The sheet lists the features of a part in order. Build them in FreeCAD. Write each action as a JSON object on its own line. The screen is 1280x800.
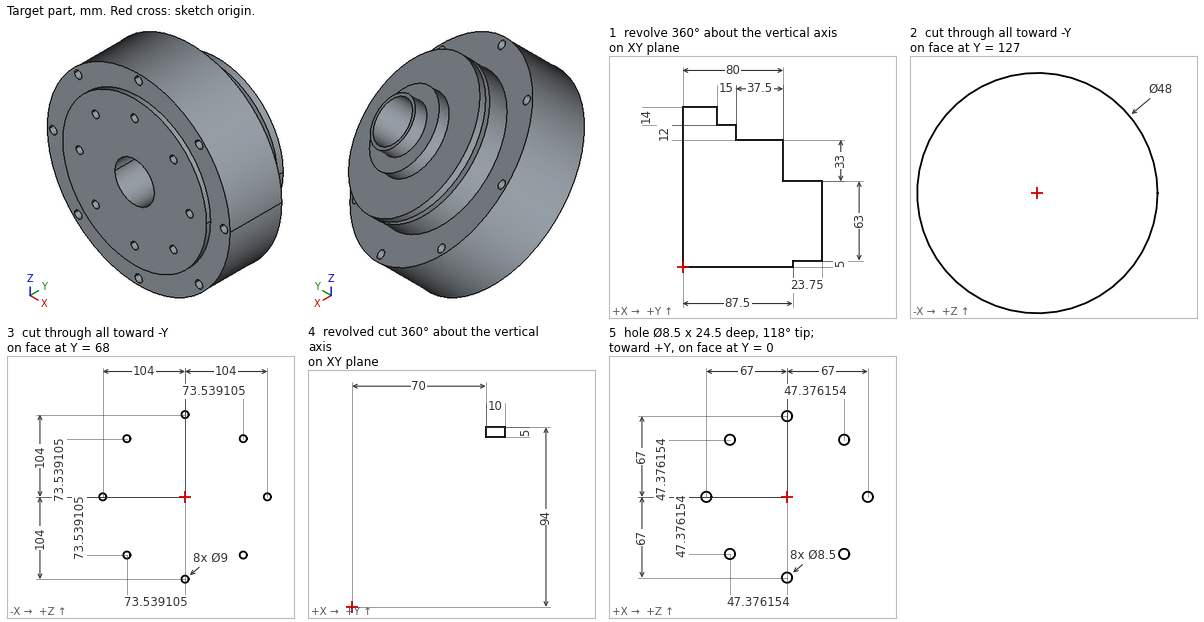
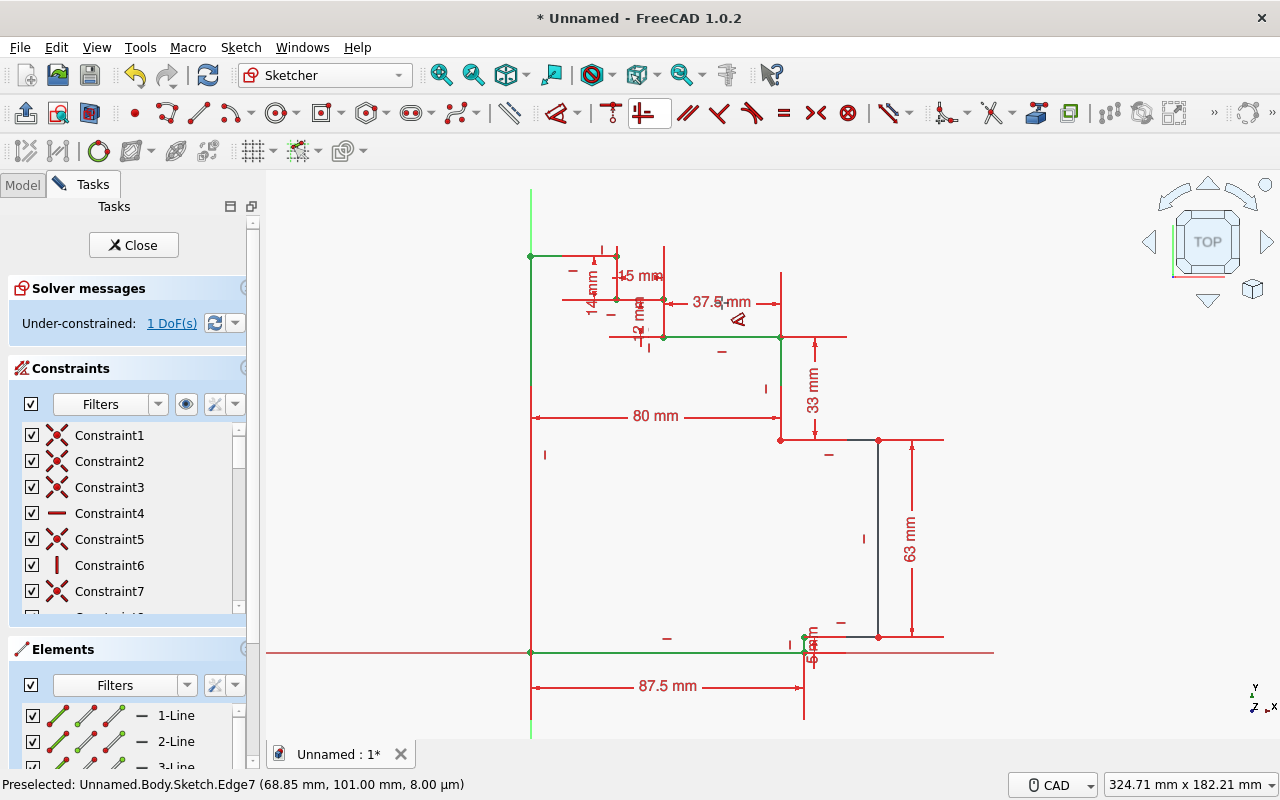
{"action": "left_click", "coordinate": [826, 637]}
{"action": "left_click", "coordinate": [841, 671]}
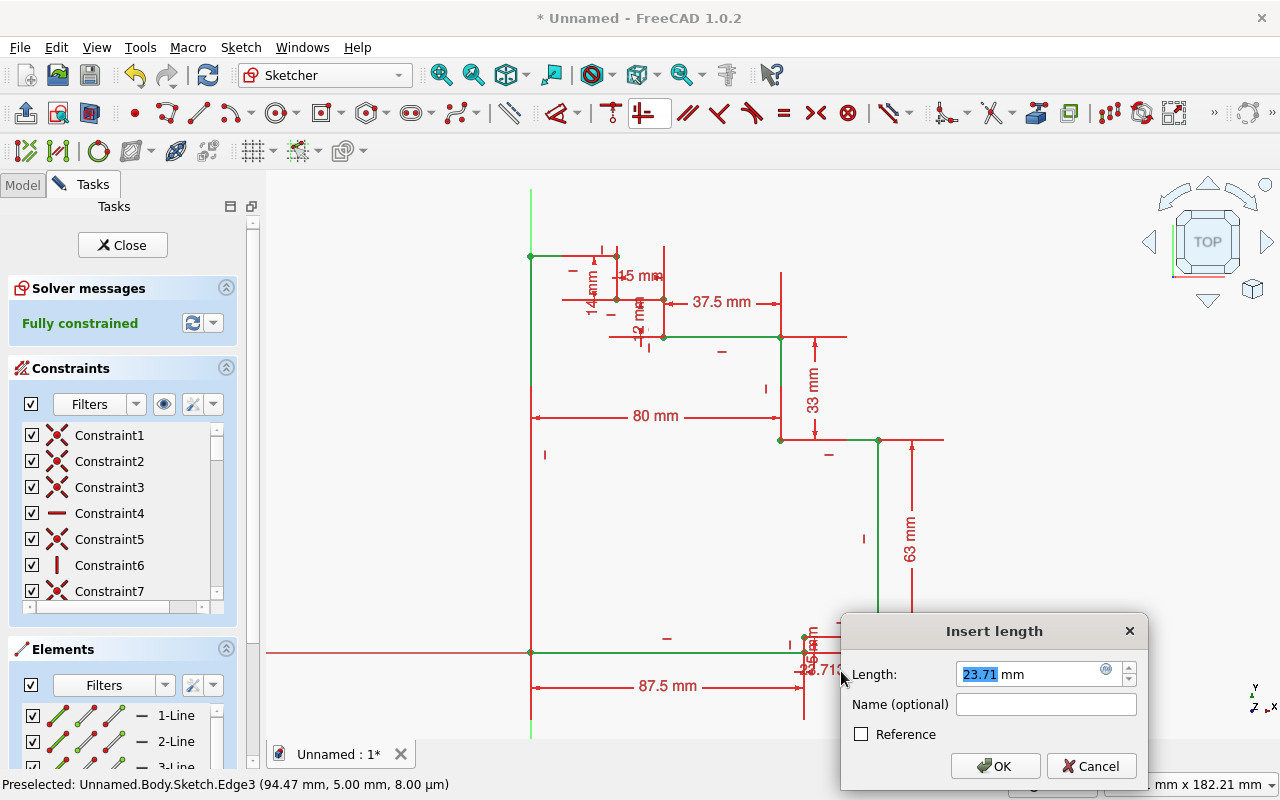
{"action": "type", "text": "23.75"}
{"action": "key", "text": "Return"}
{"action": "key", "text": "Escape"}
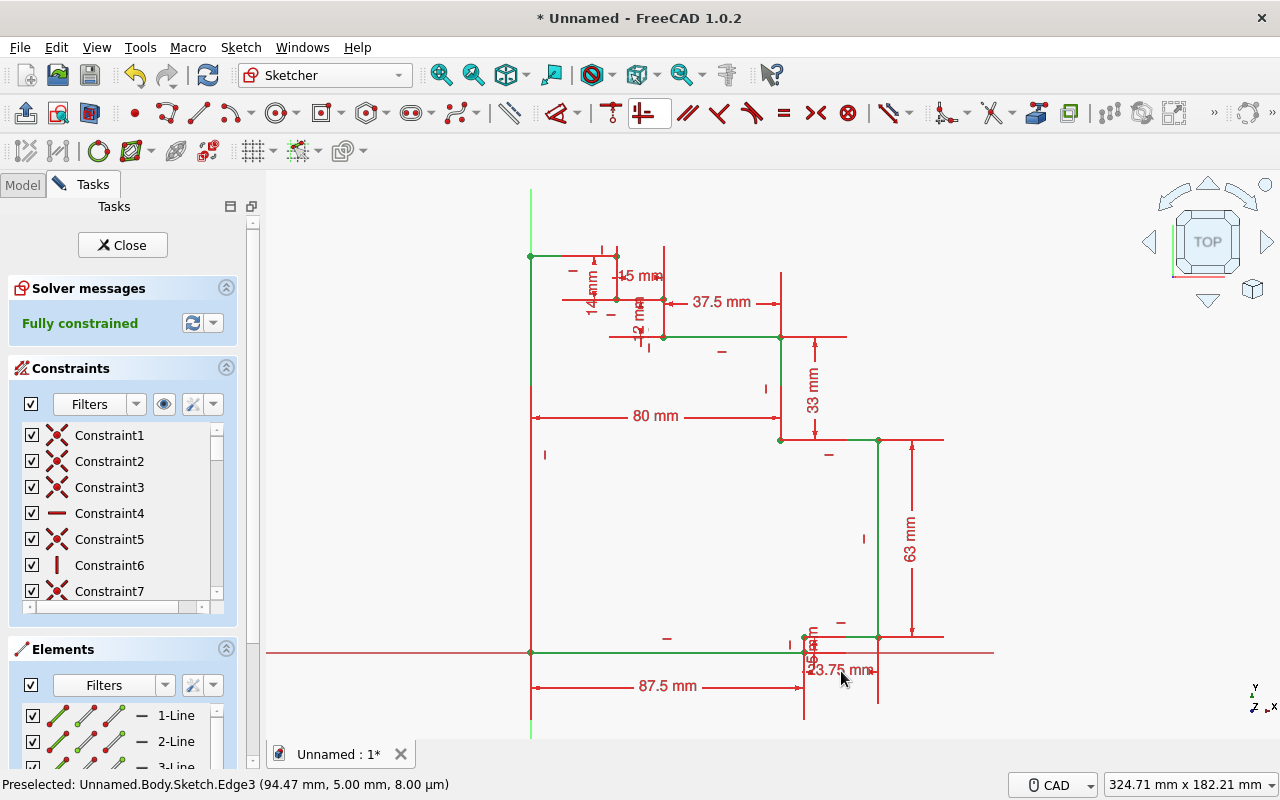
{"action": "left_click", "coordinate": [123, 245]}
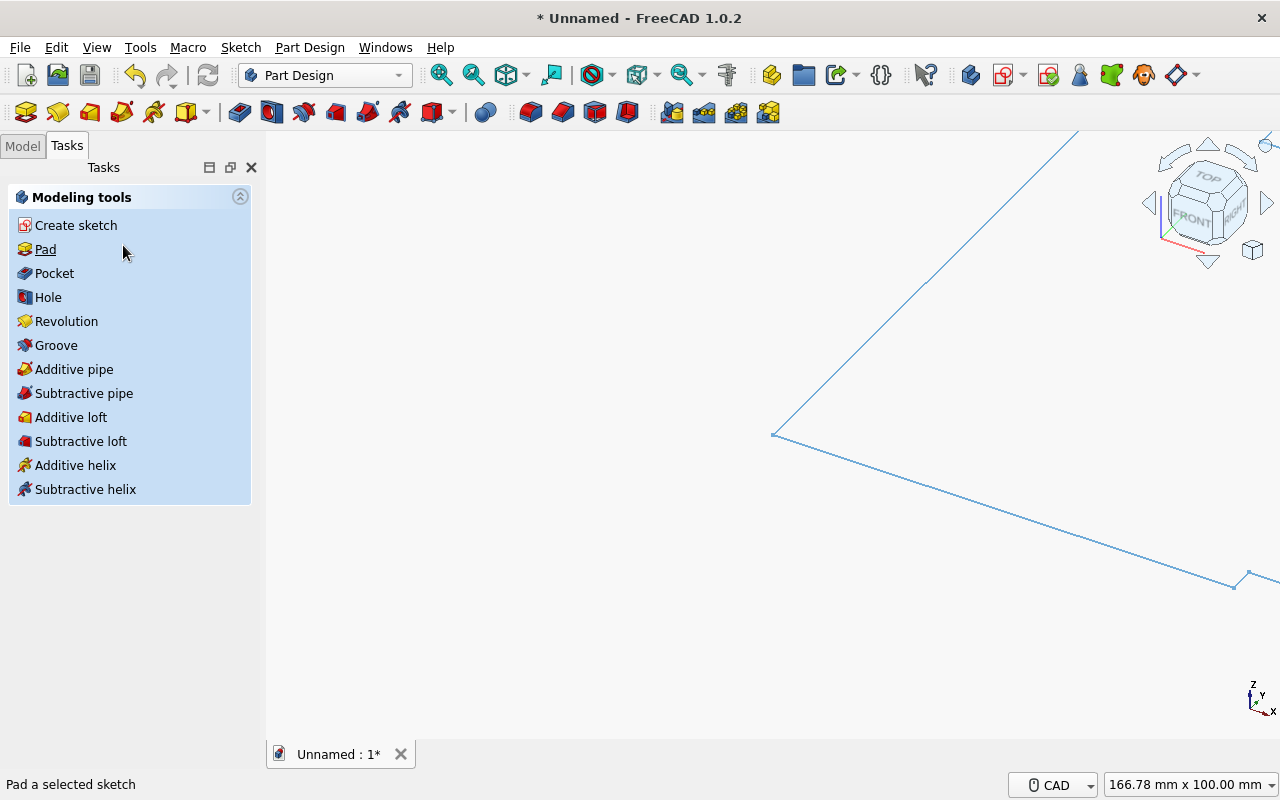
{"action": "left_click", "coordinate": [58, 112]}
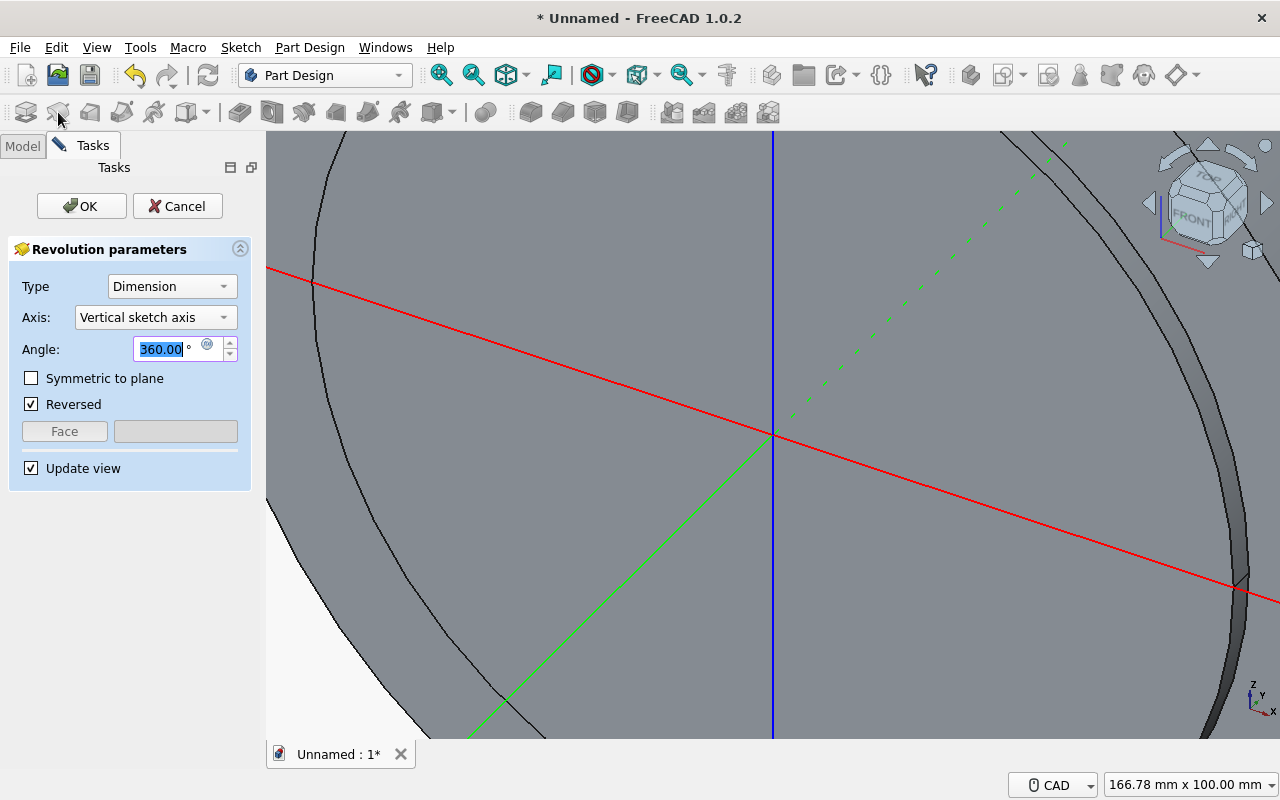
{"action": "left_click", "coordinate": [82, 206]}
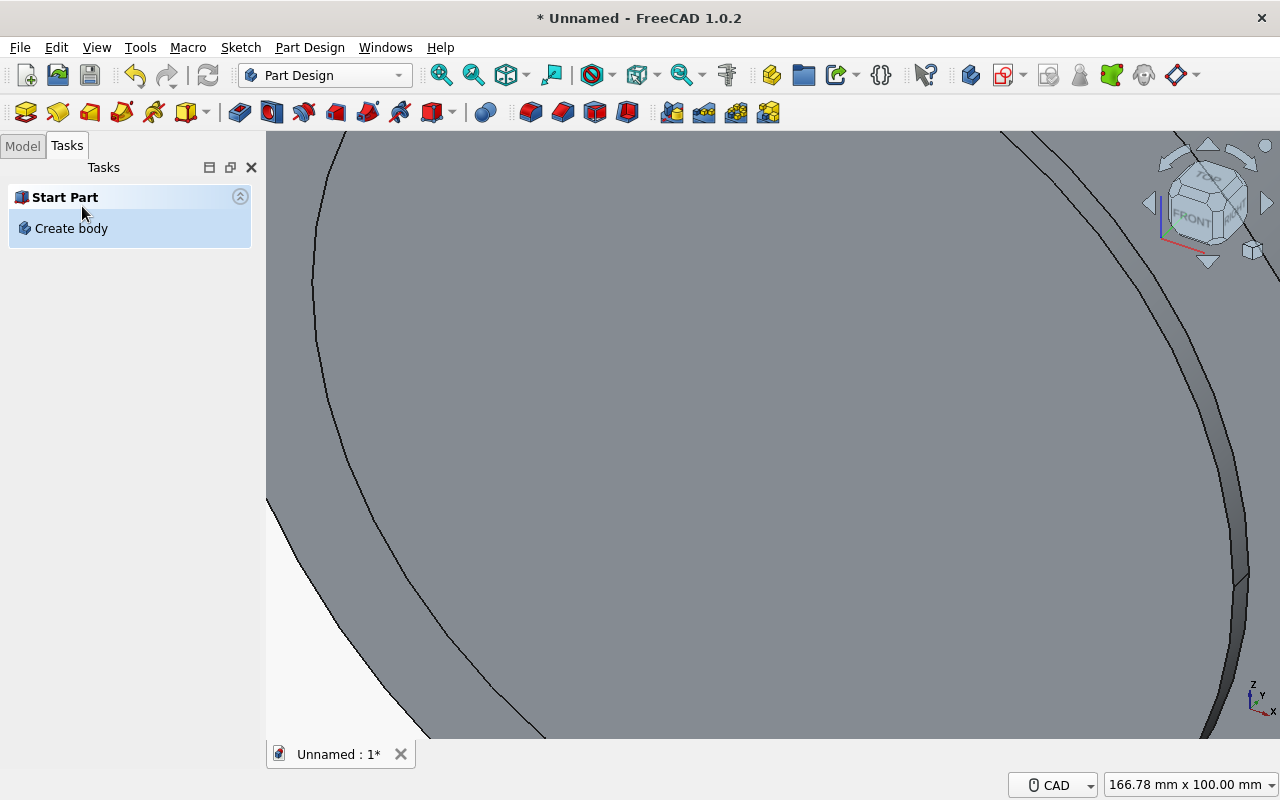
{"action": "left_click", "coordinate": [442, 76]}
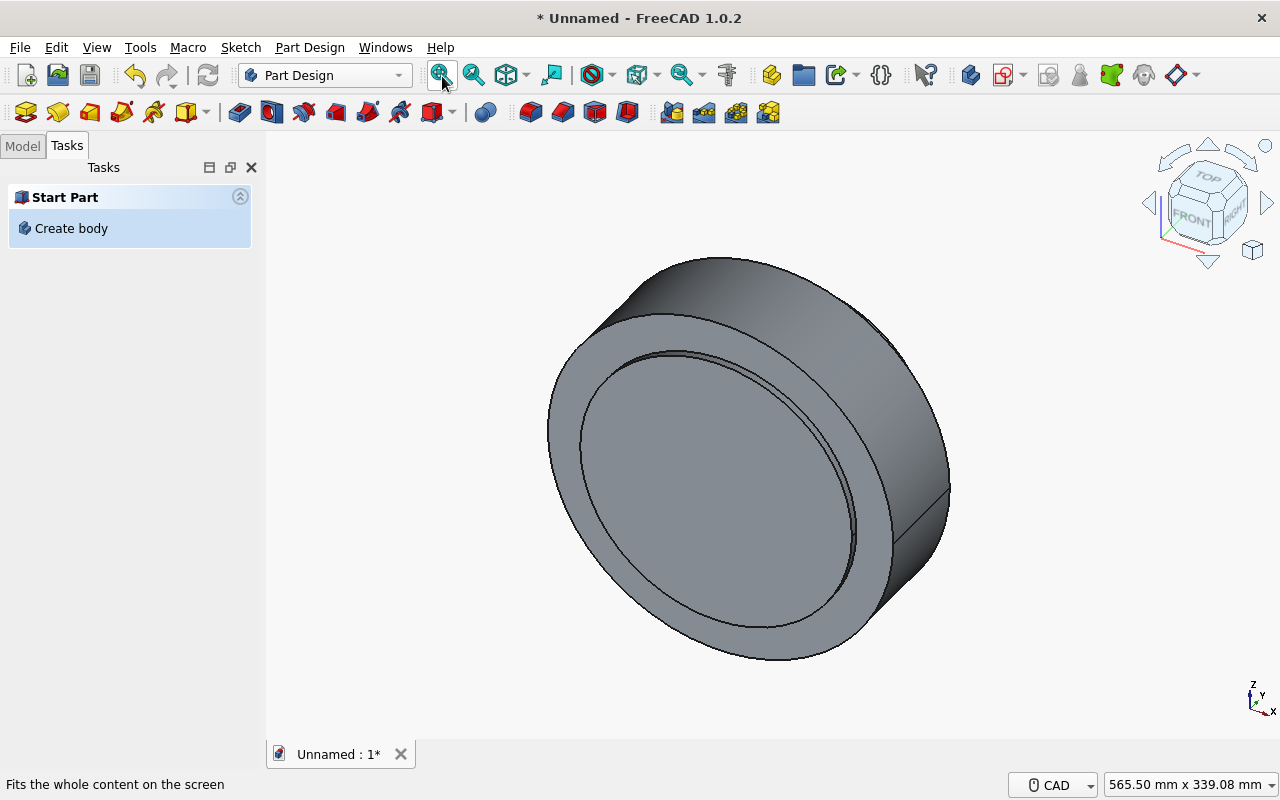
{"action": "key", "text": "4"}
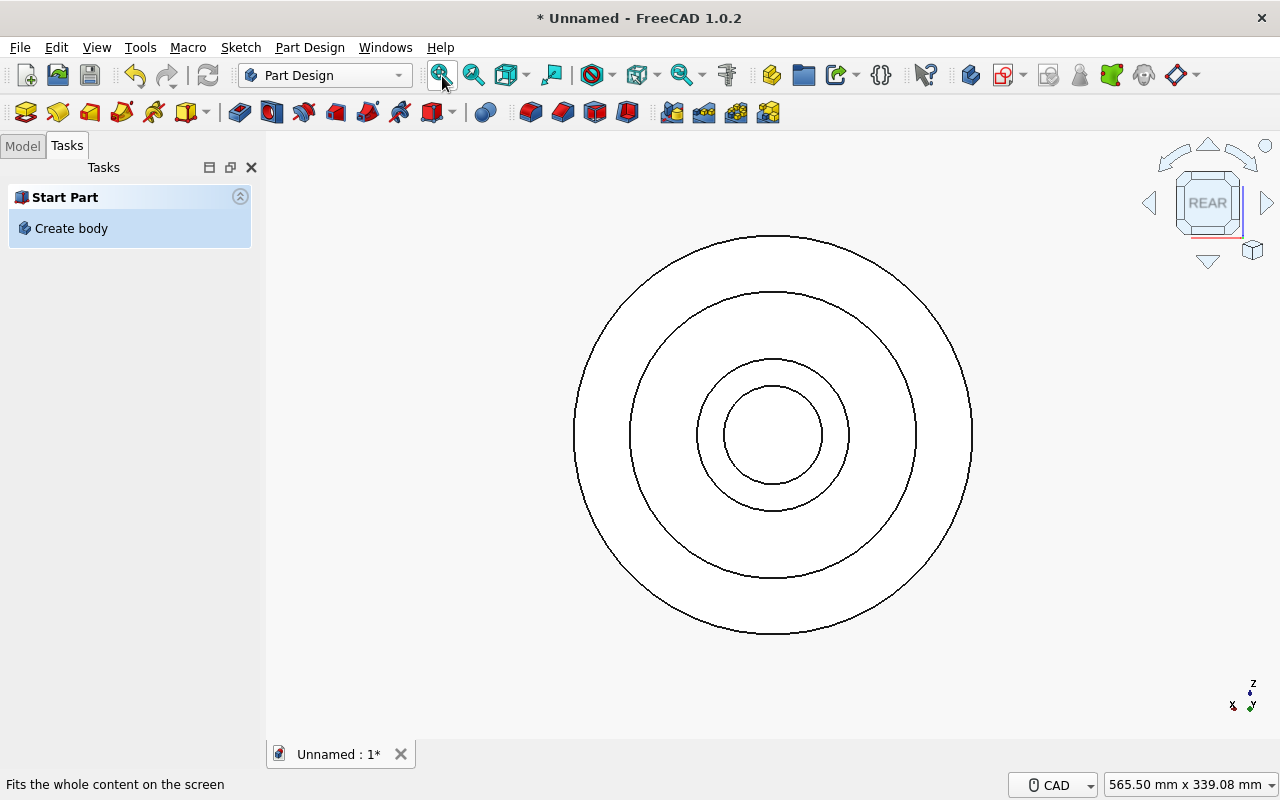
{"action": "left_click", "coordinate": [773, 434]}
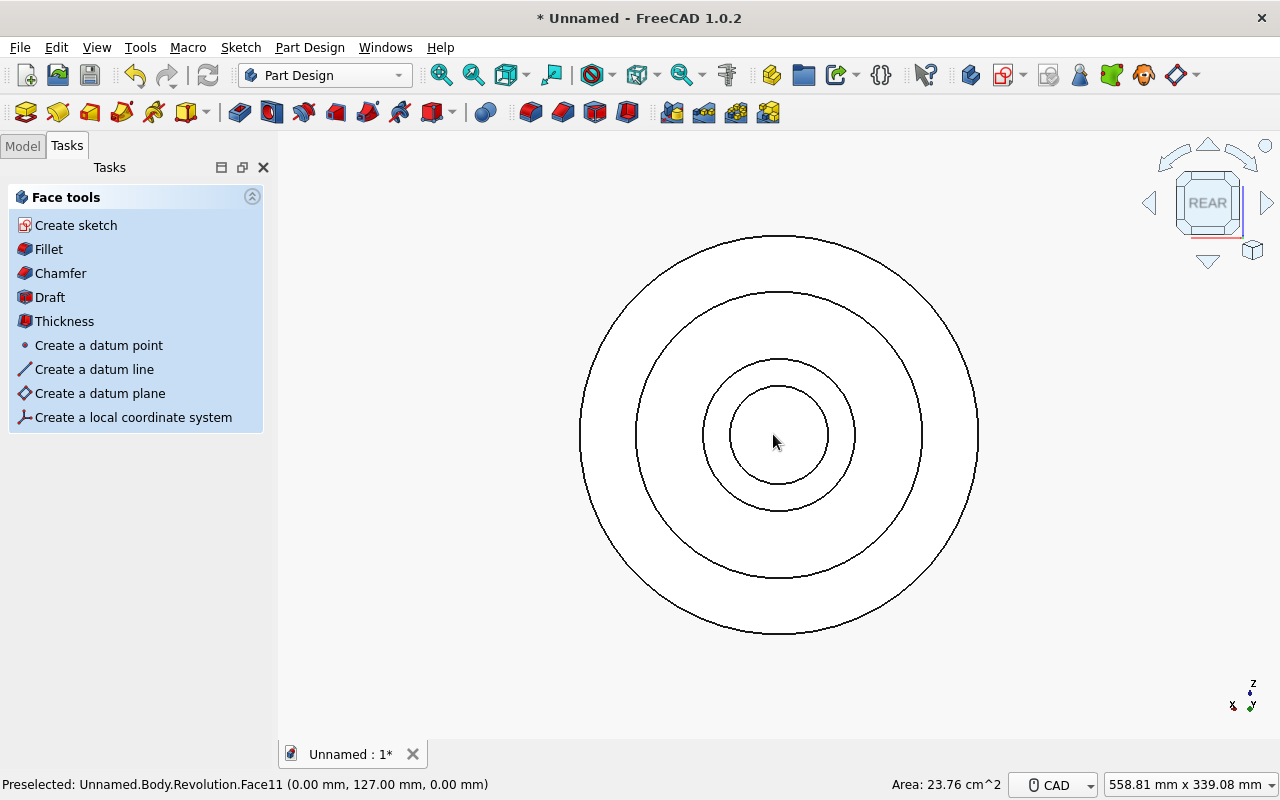
{"action": "left_click", "coordinate": [1004, 76]}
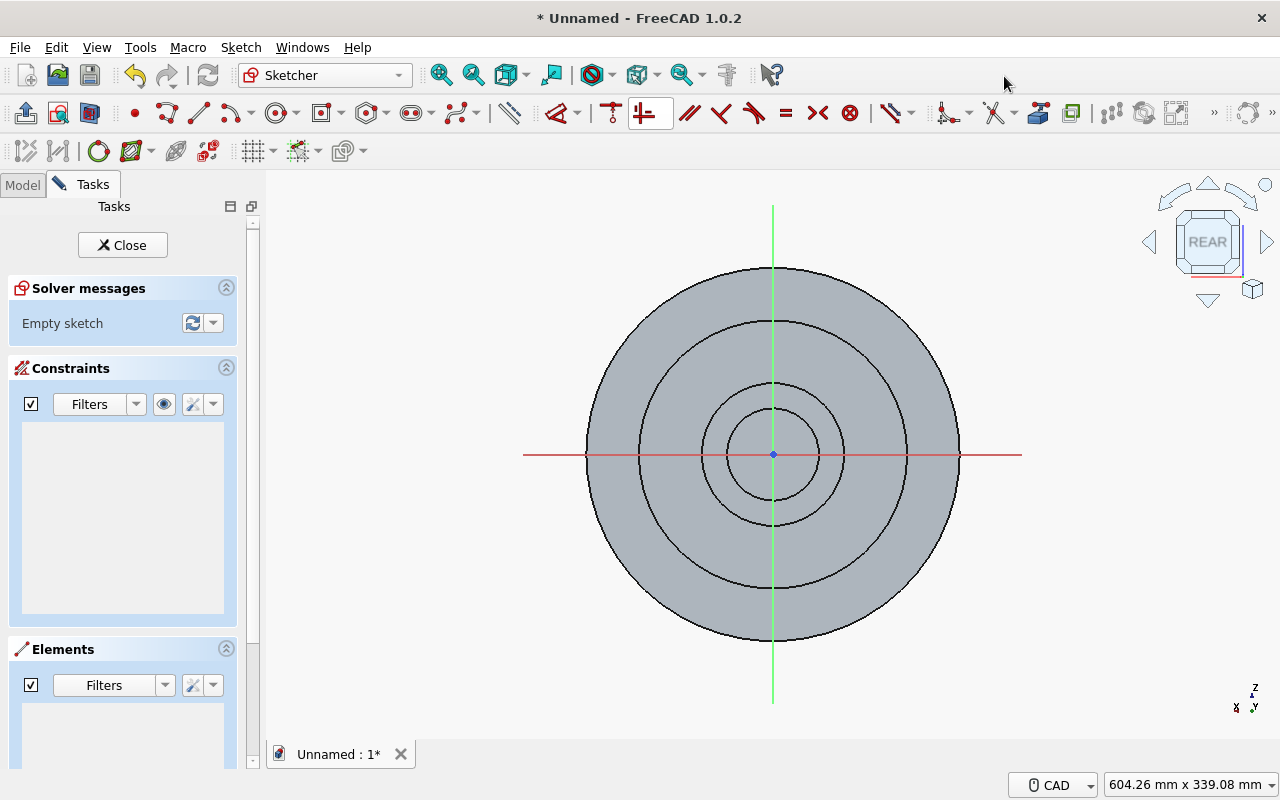
{"action": "scroll", "coordinate": [790, 454], "scroll_direction": "up", "scroll_amount": 8}